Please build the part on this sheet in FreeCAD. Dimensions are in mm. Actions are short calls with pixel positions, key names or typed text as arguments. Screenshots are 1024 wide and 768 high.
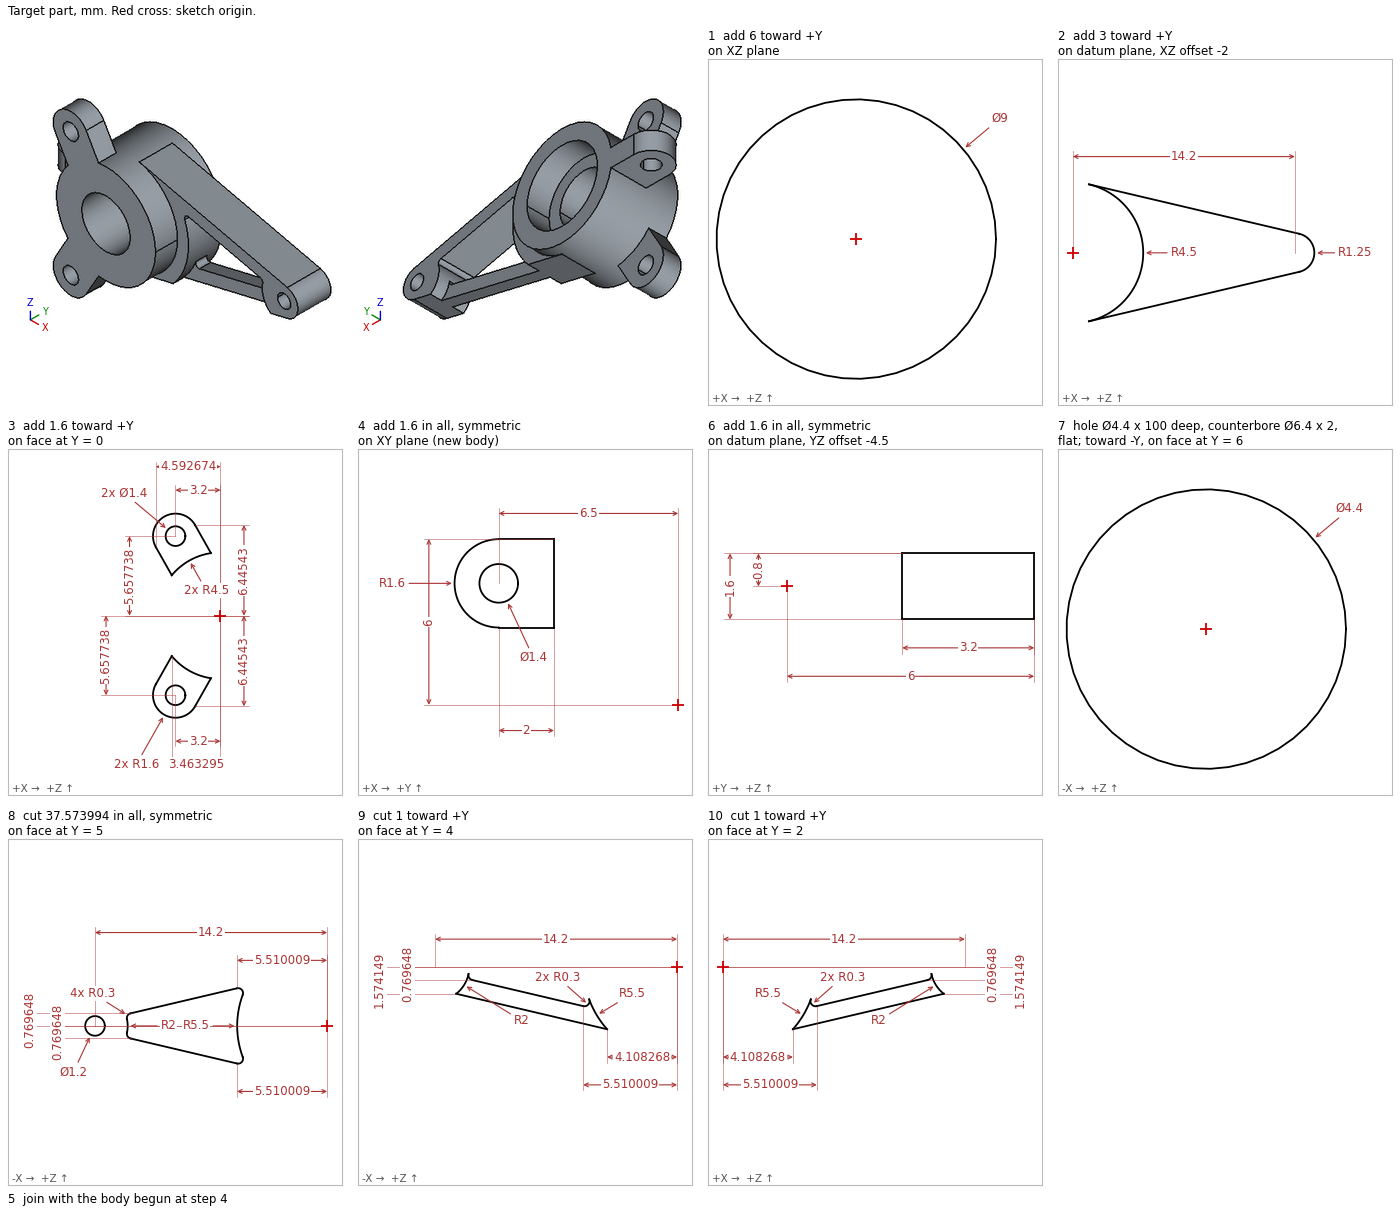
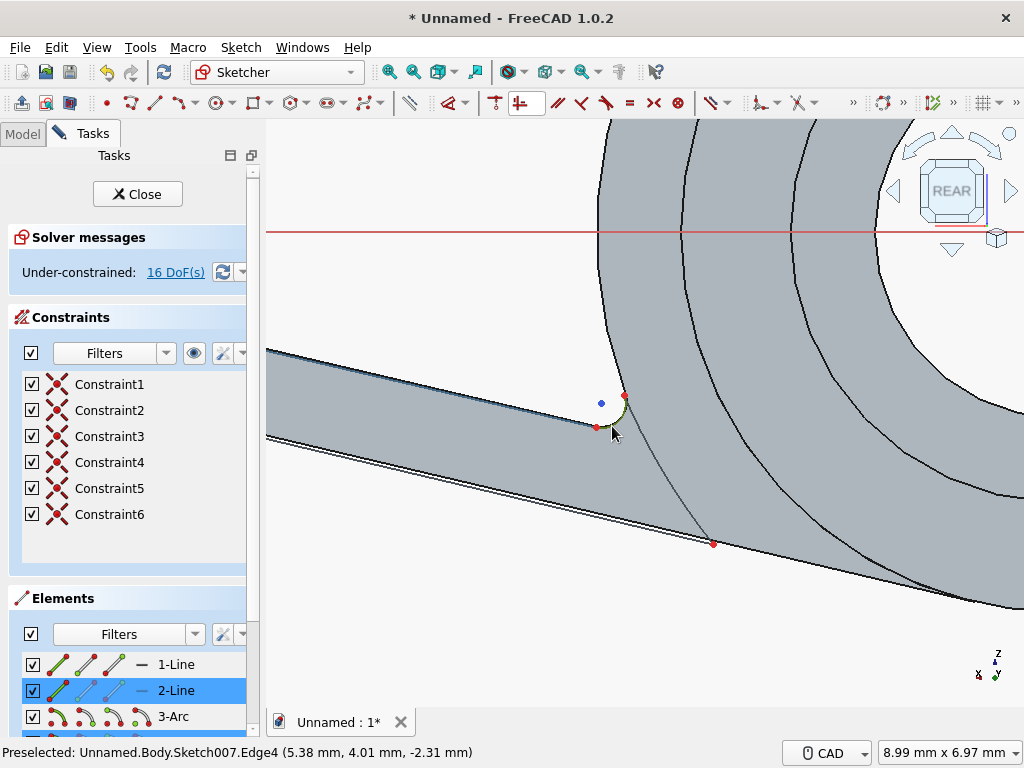
key(t)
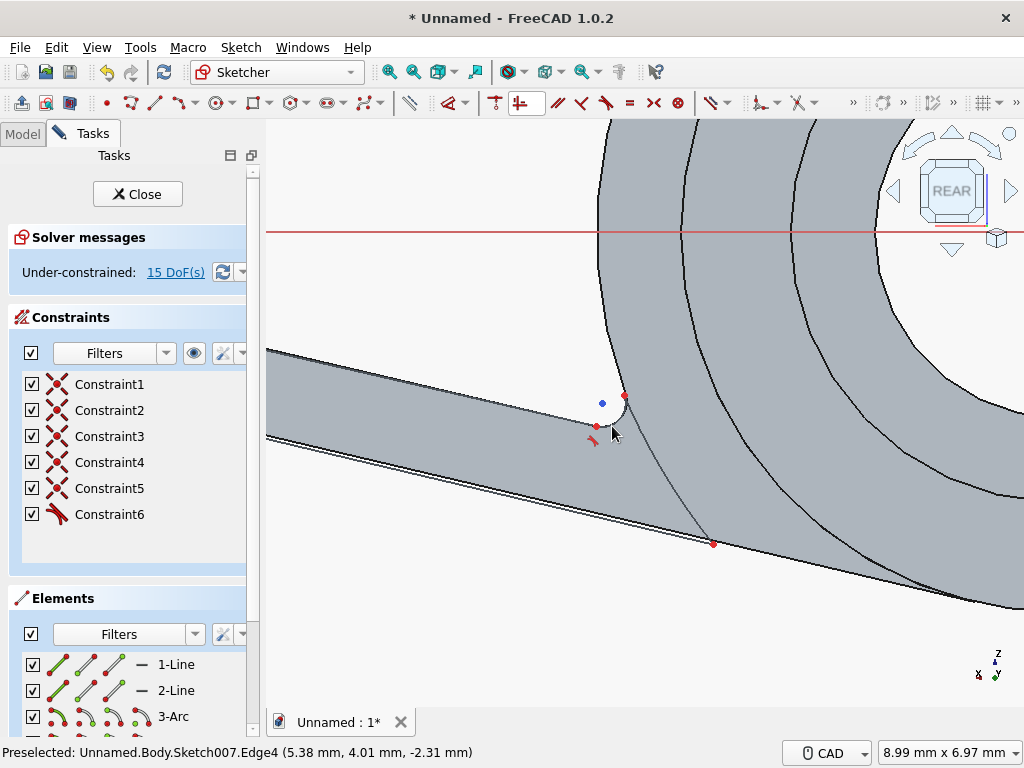
click(432, 389)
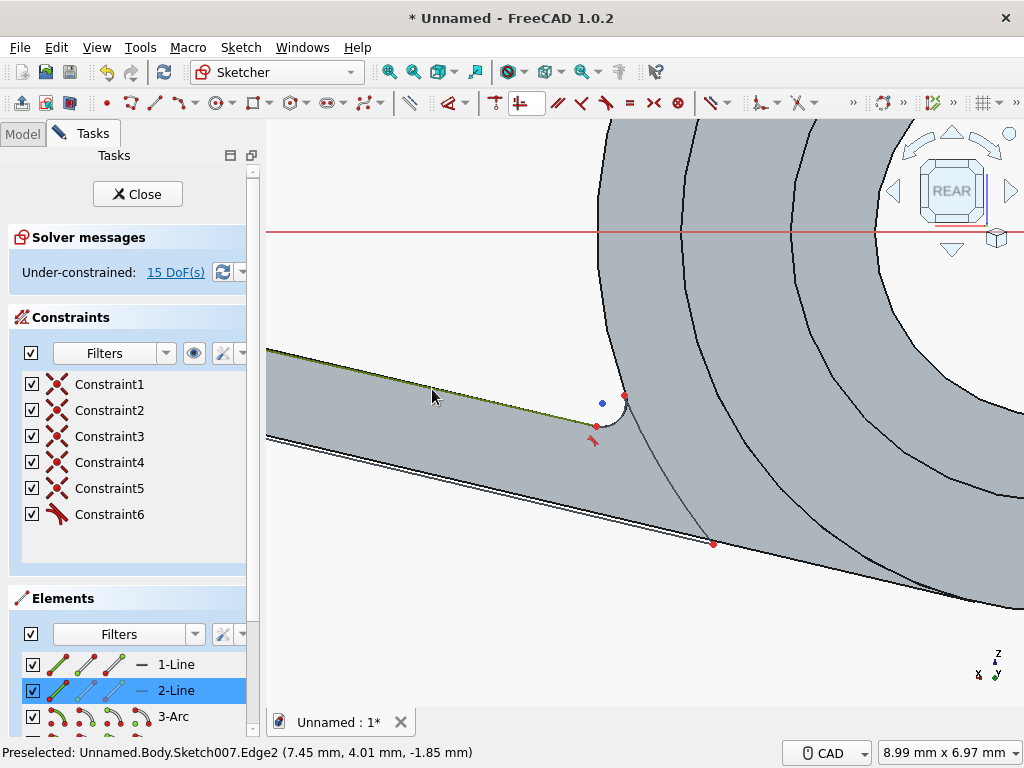
scroll(613, 428, down, 5)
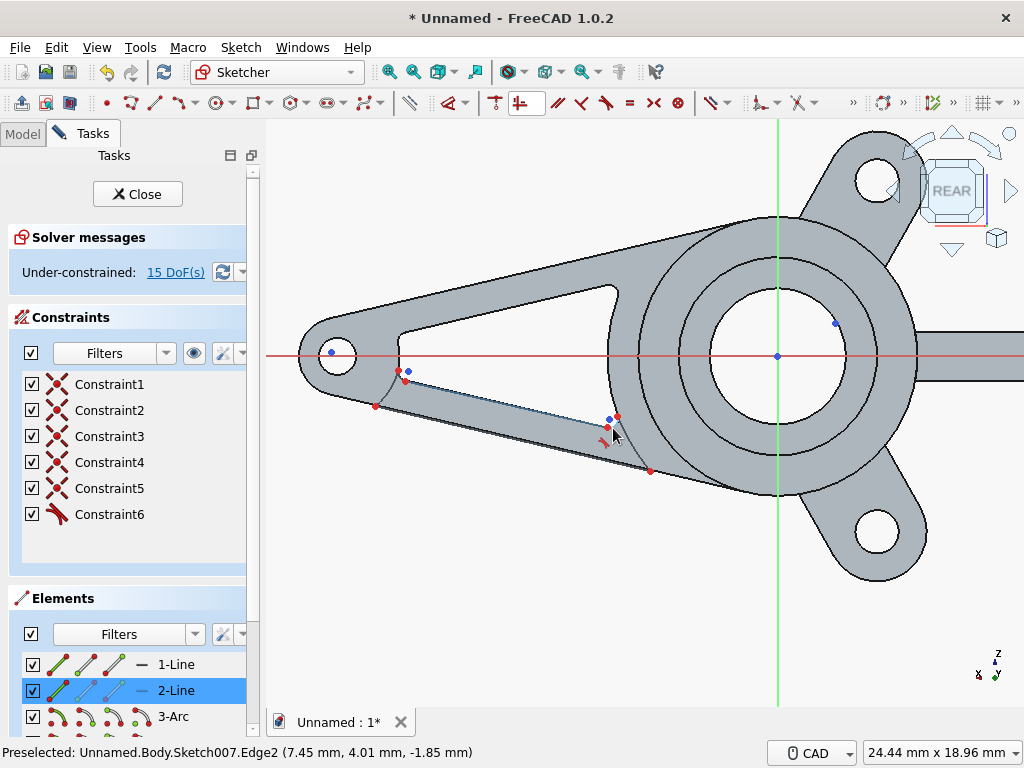
scroll(402, 379, up, 6)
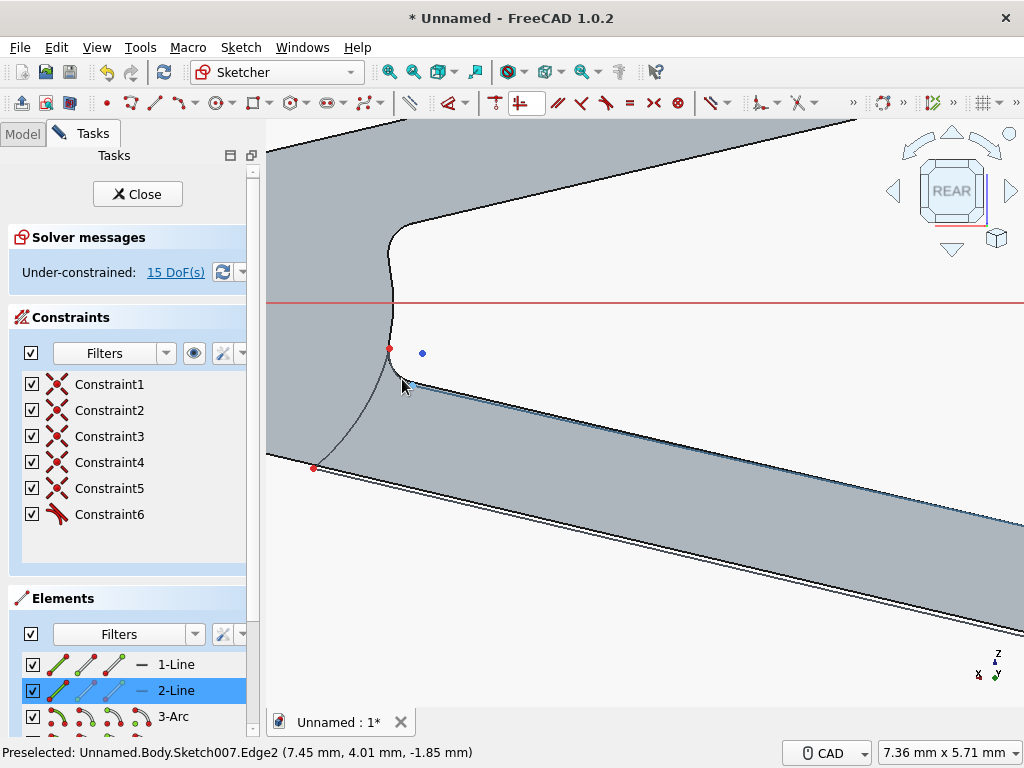
click(400, 379)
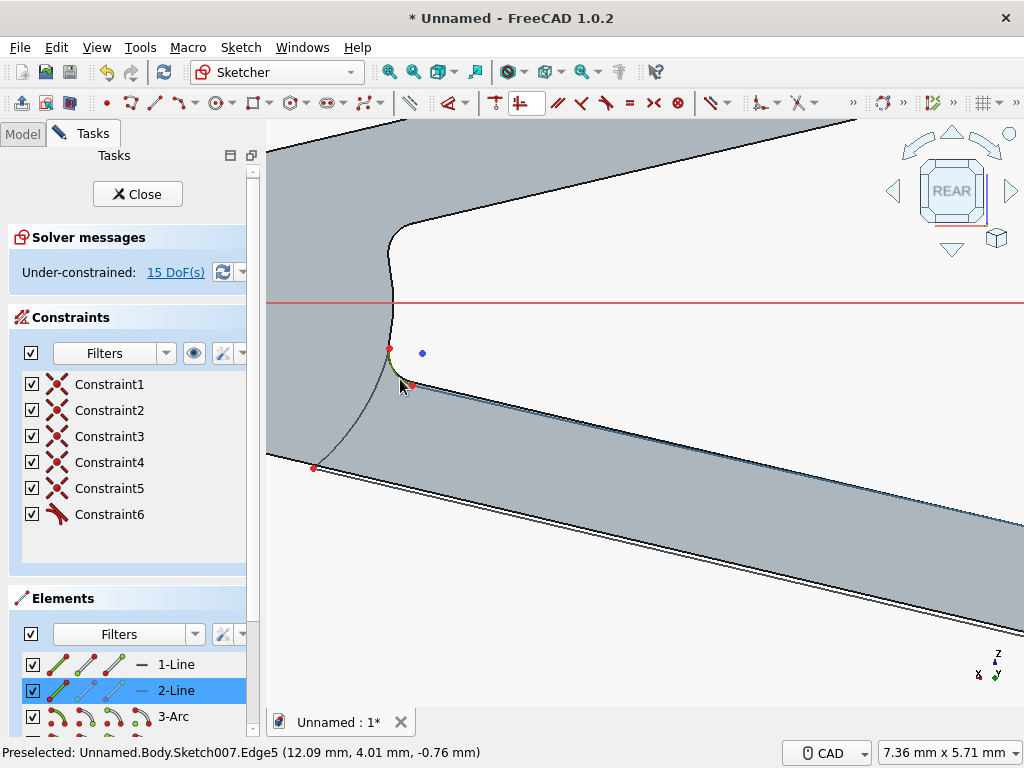
key(t)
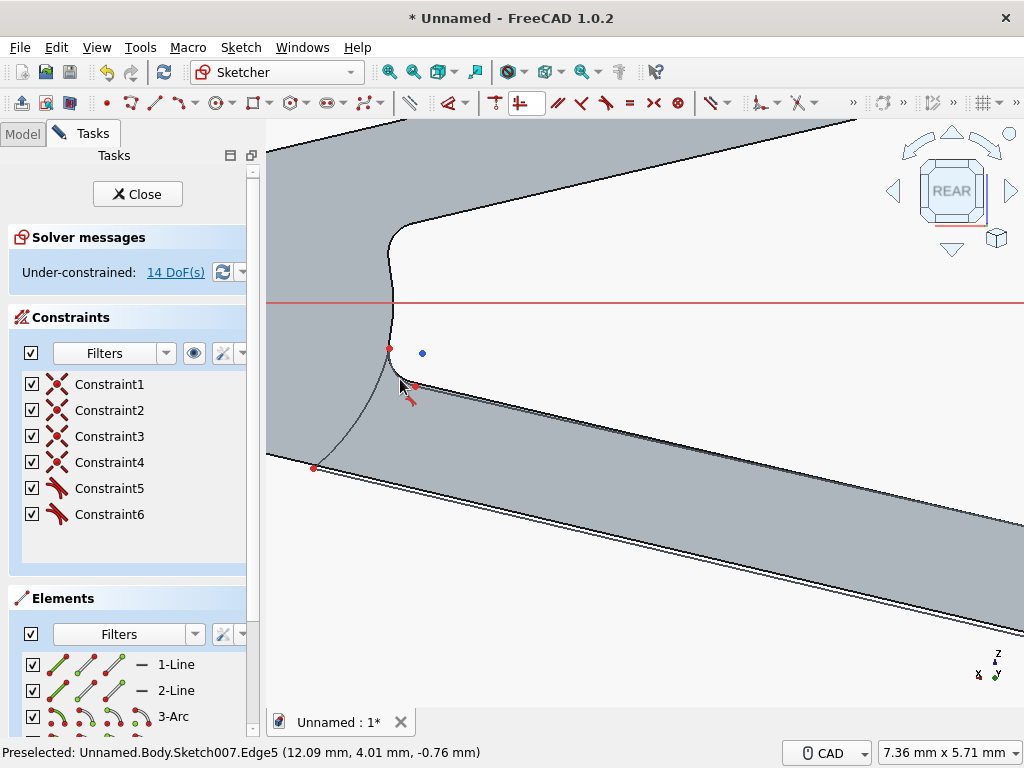
scroll(402, 379, down, 6)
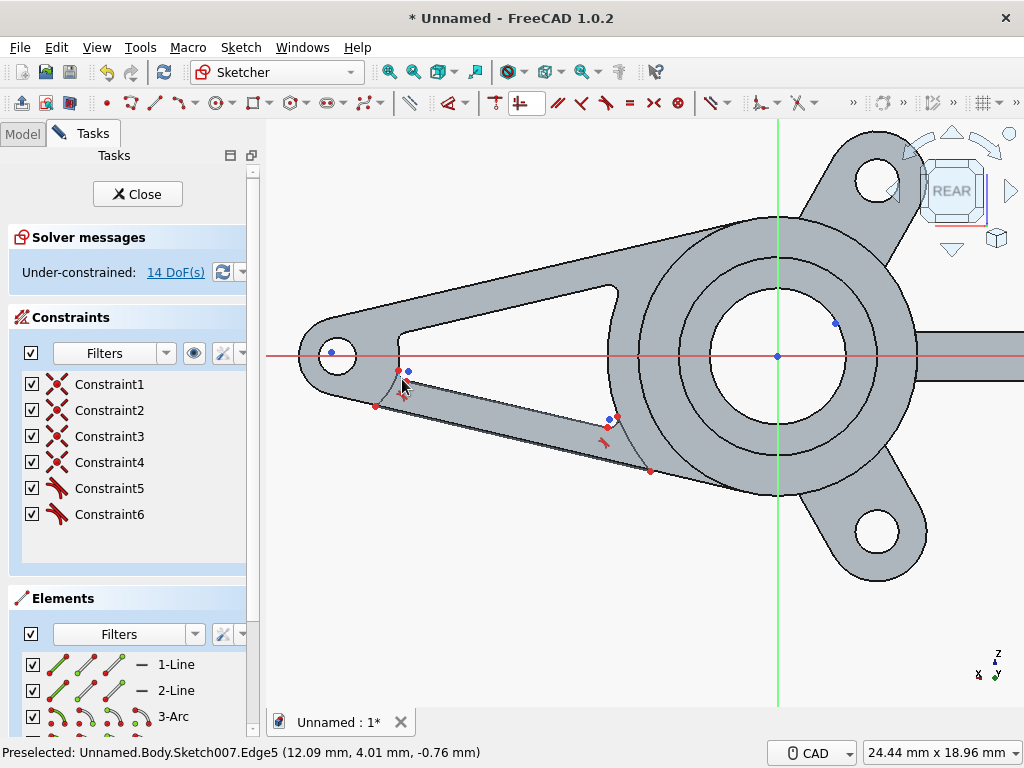
click(626, 434)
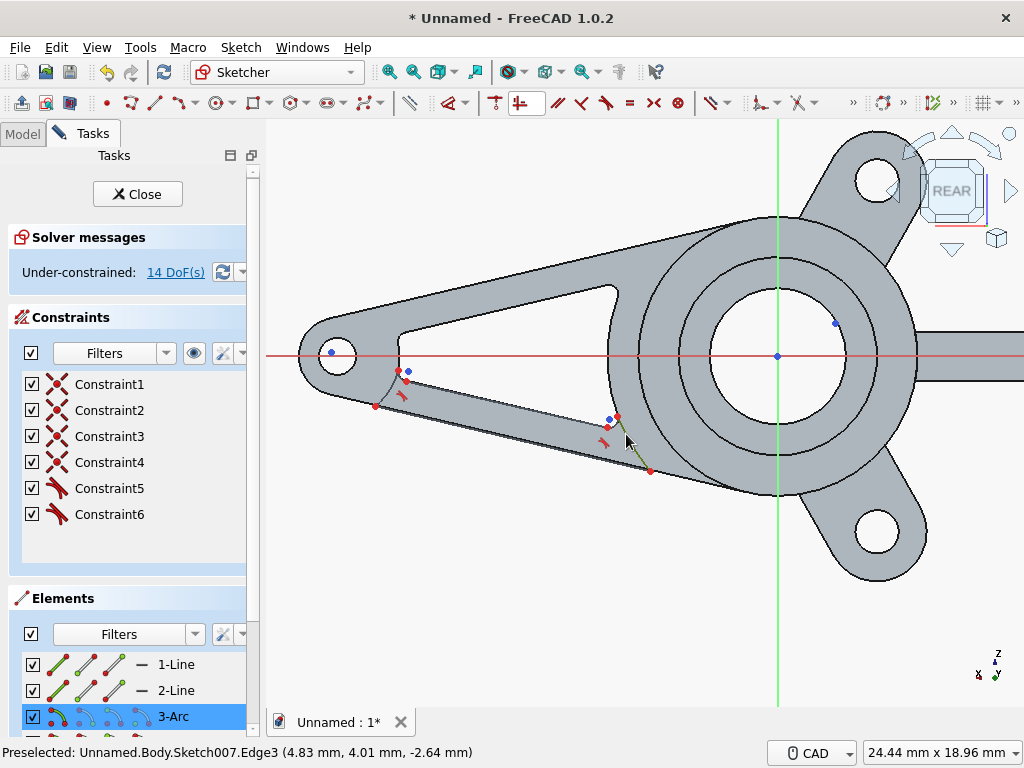
scroll(613, 427, up, 5)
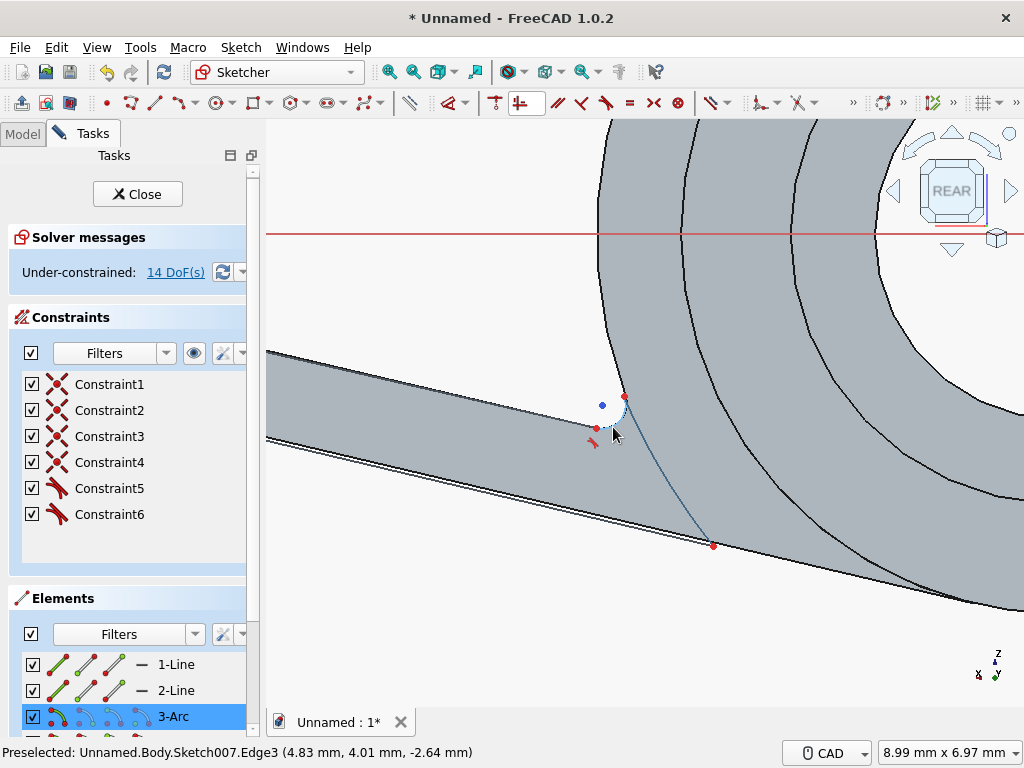
click(612, 427)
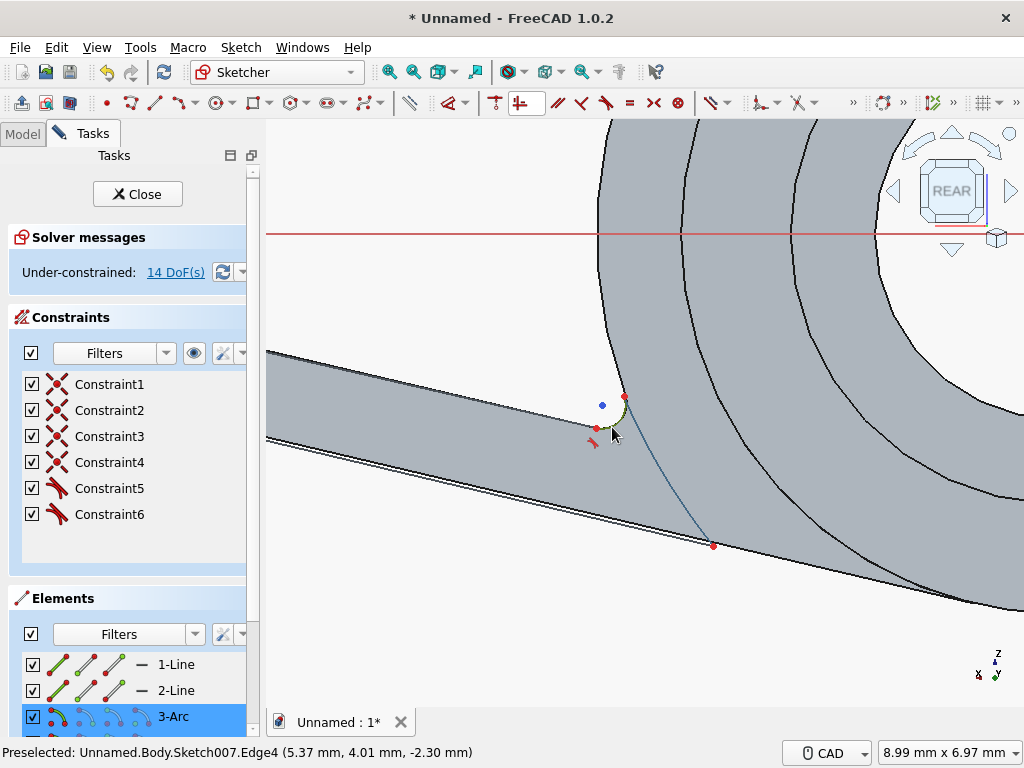
click(606, 104)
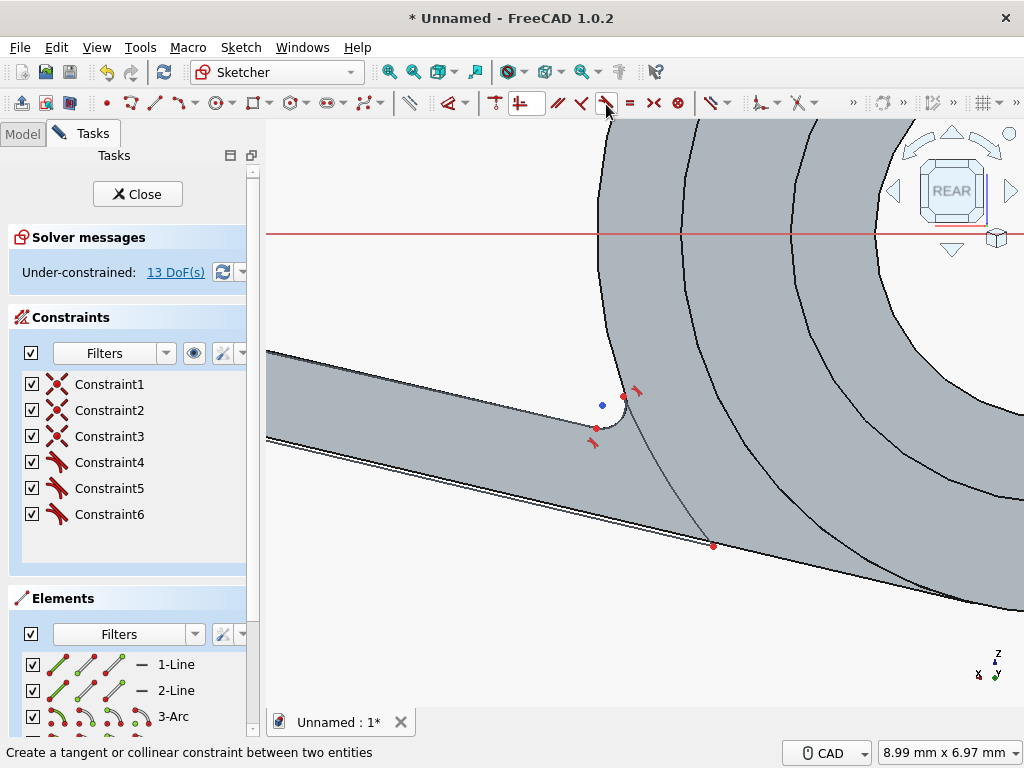
scroll(613, 427, down, 5)